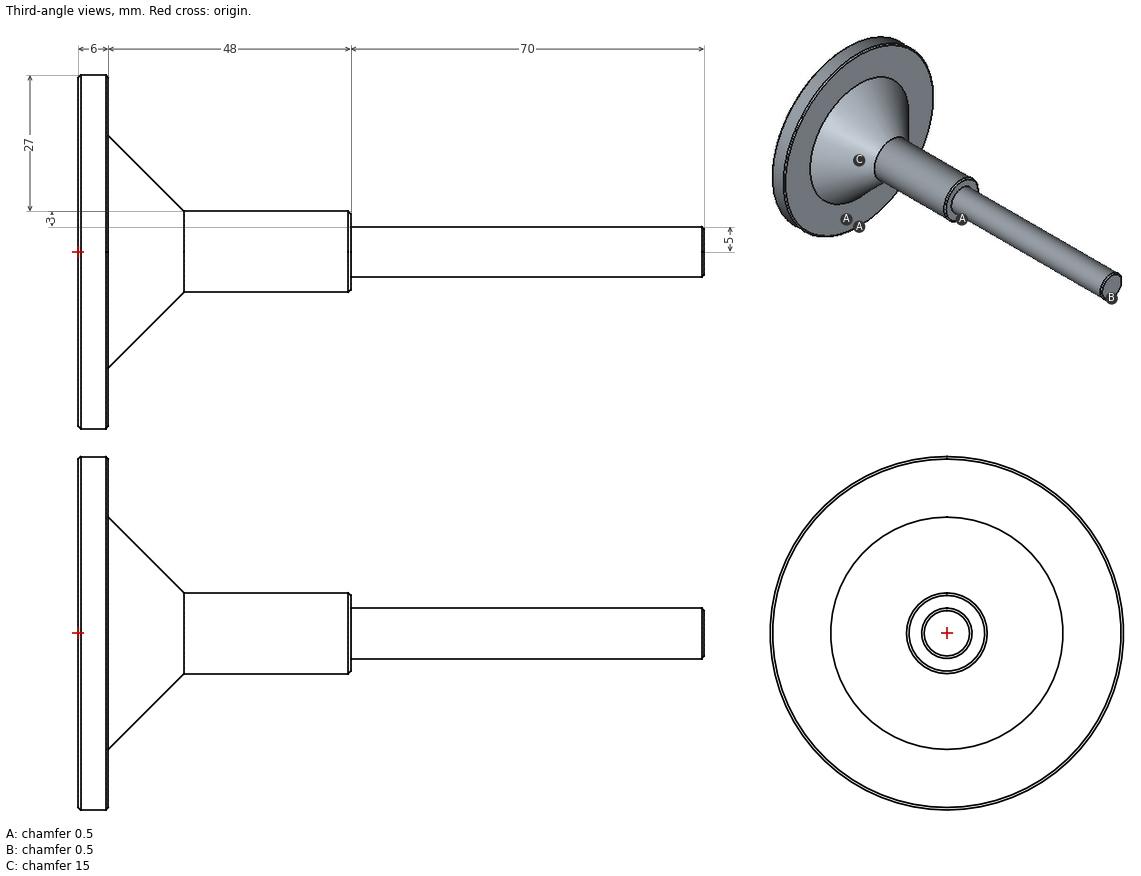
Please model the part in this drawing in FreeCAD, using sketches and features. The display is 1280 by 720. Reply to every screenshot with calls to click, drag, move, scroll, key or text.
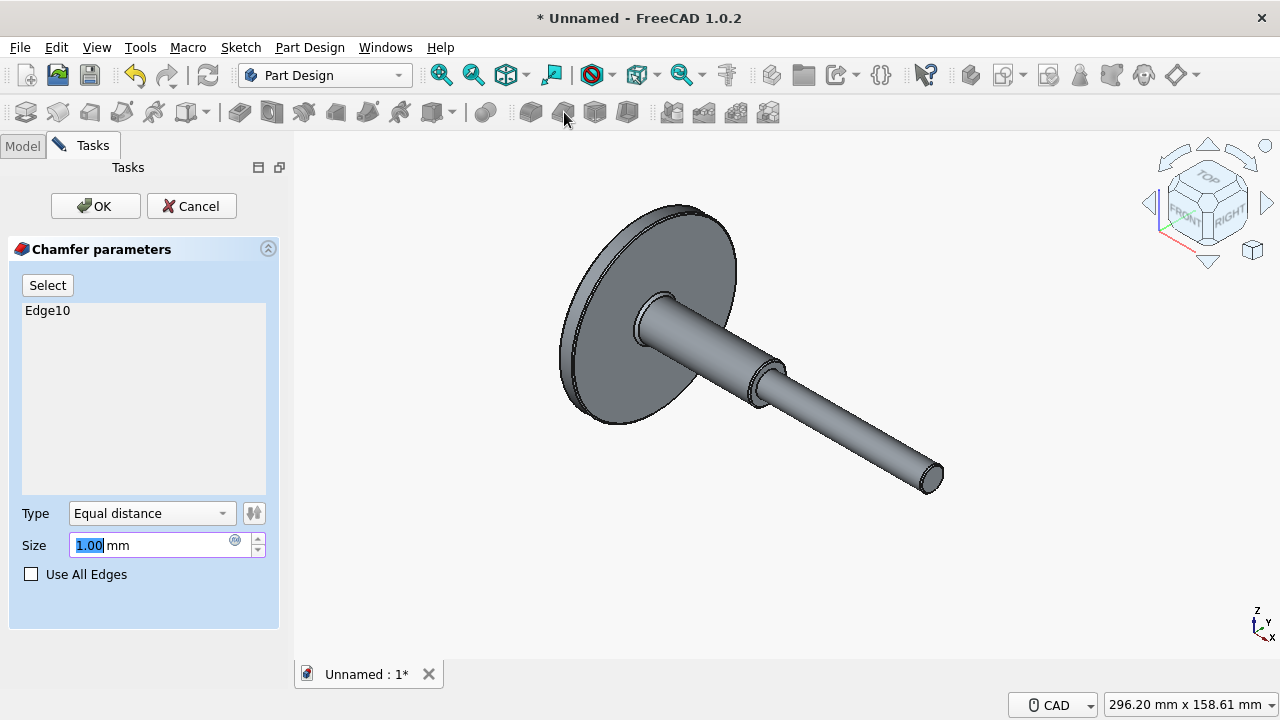
text(15)
key(Tab)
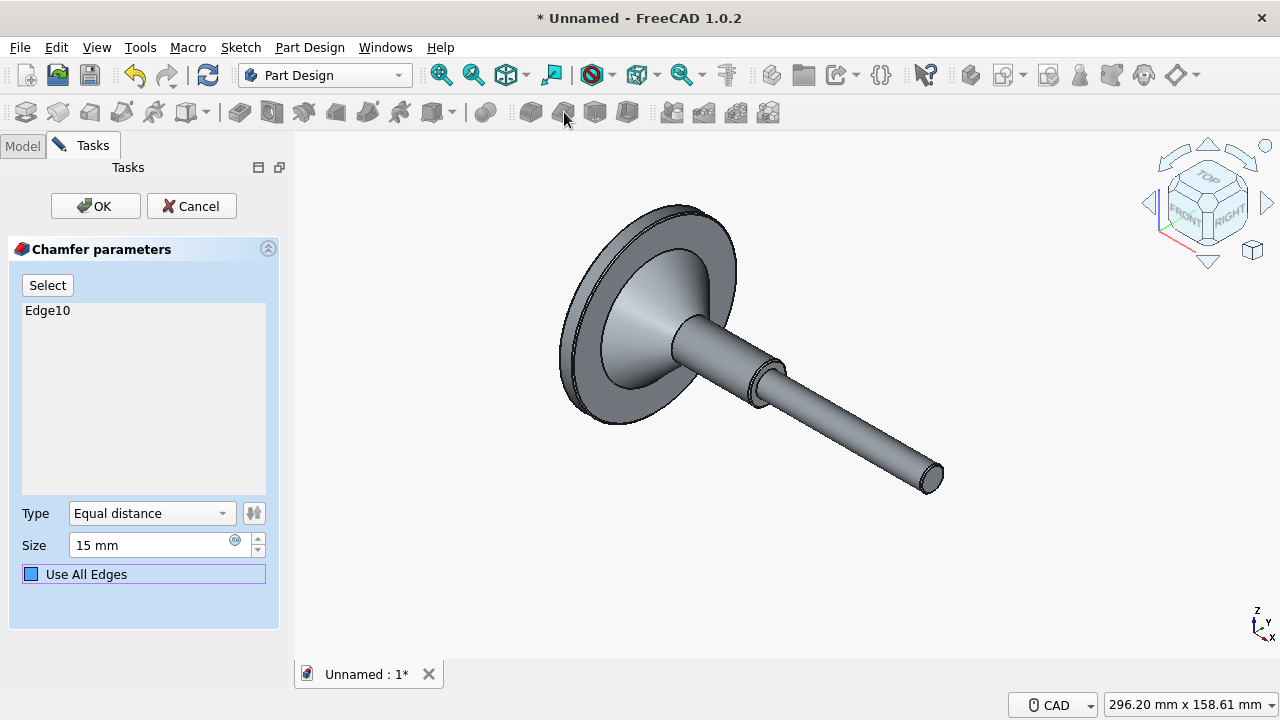
click(96, 206)